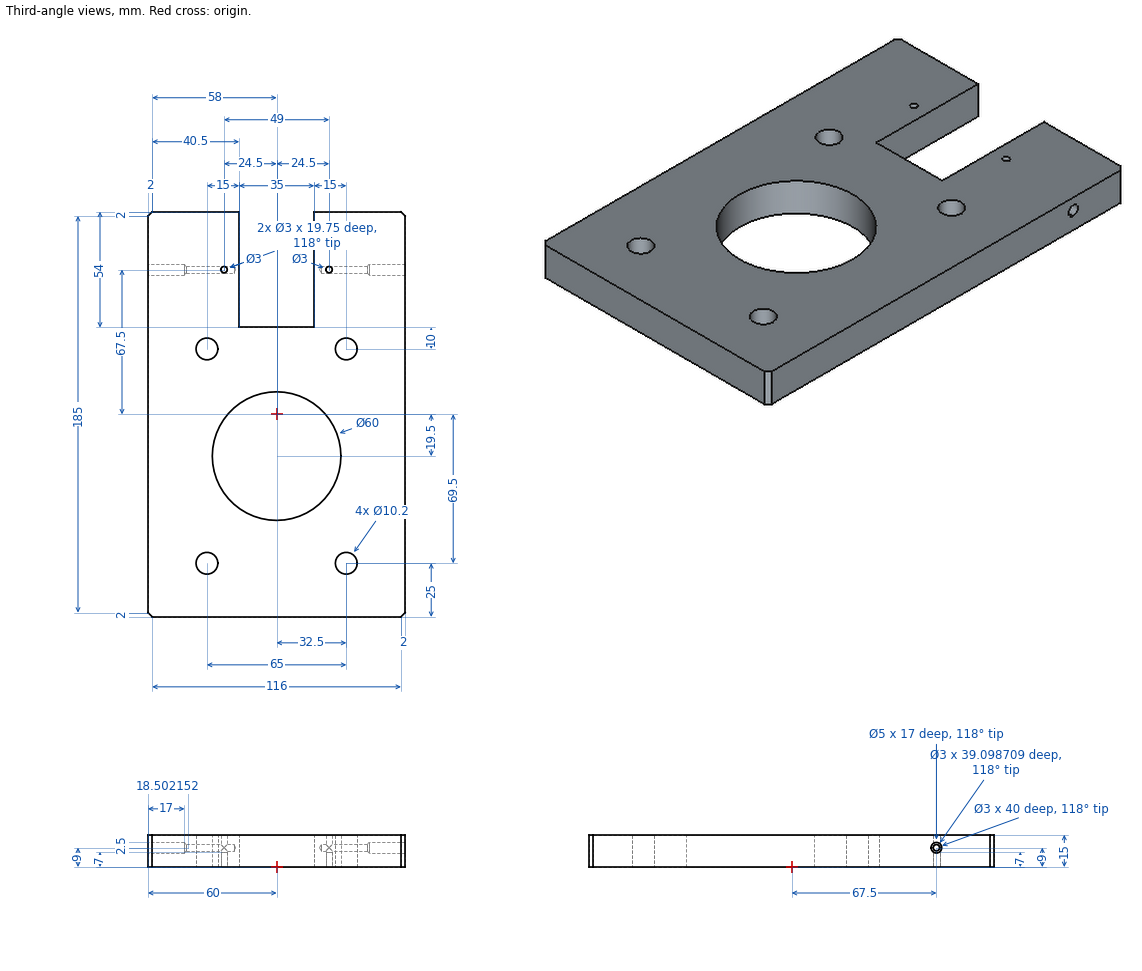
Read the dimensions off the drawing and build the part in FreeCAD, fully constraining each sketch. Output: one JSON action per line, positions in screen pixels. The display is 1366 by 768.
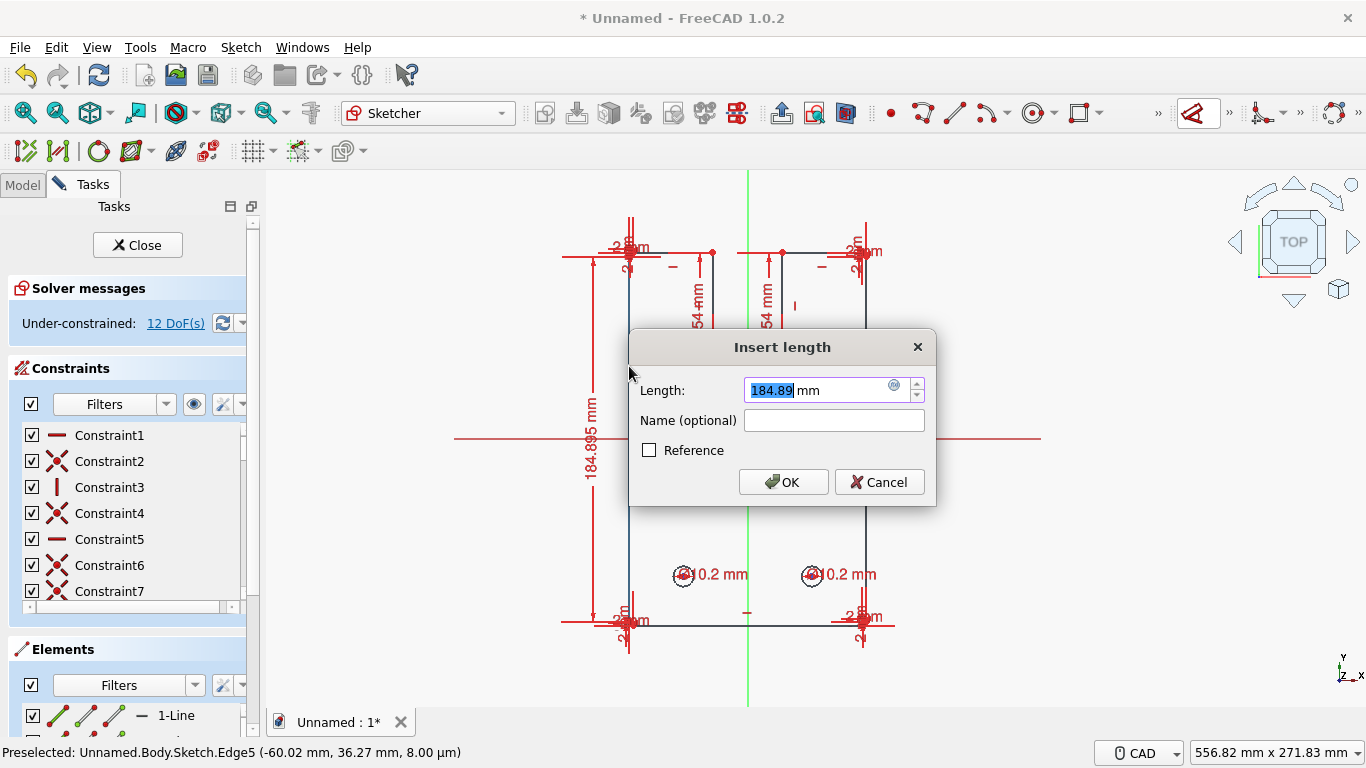
{"action": "type", "text": "185"}
{"action": "key", "text": "Return"}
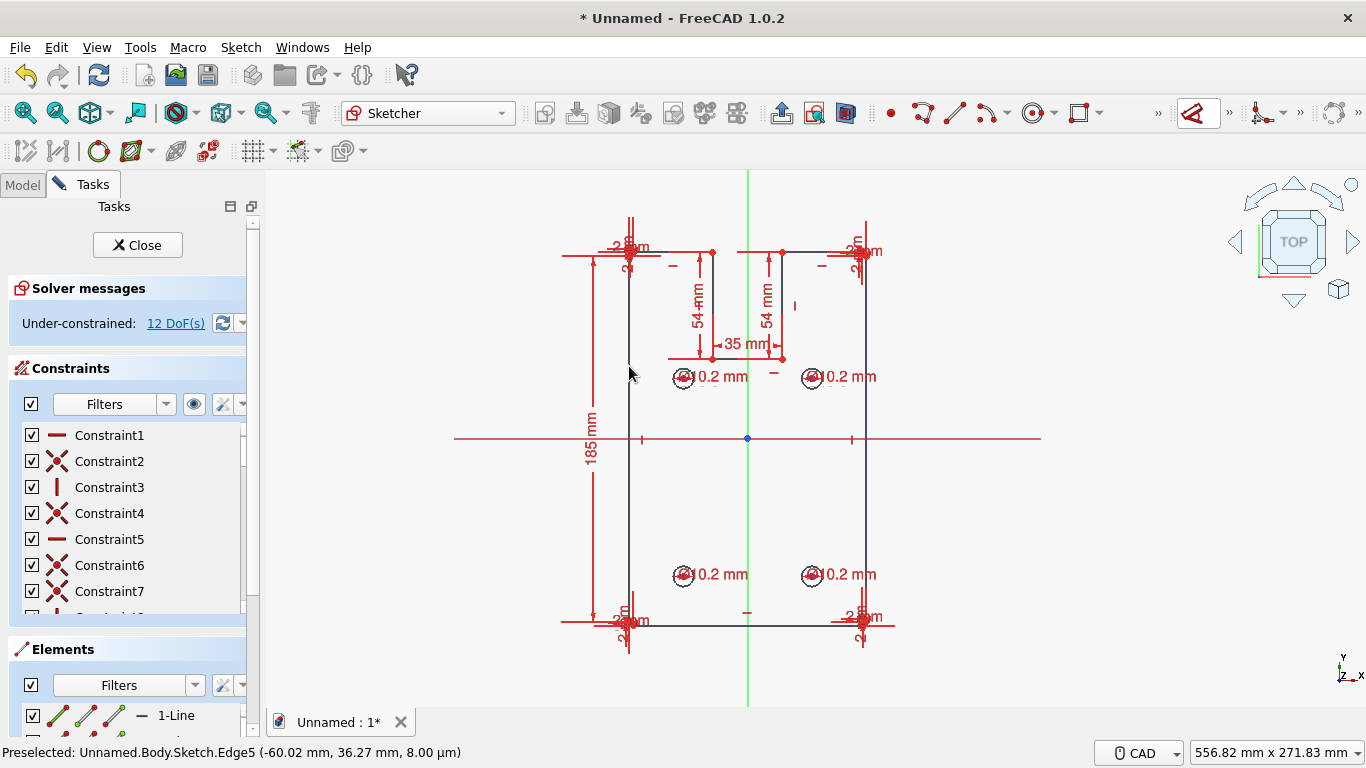
{"action": "left_click", "coordinate": [702, 626]}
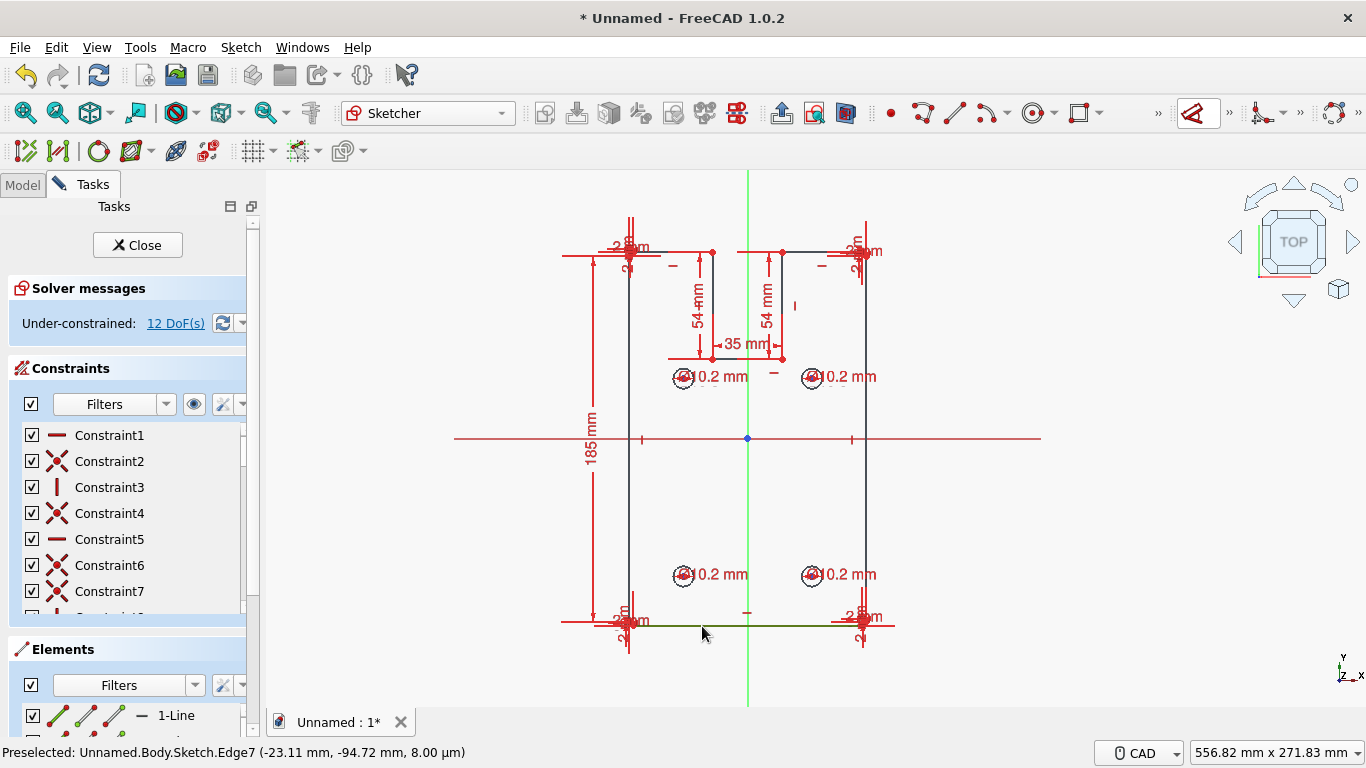
{"action": "key", "text": "l"}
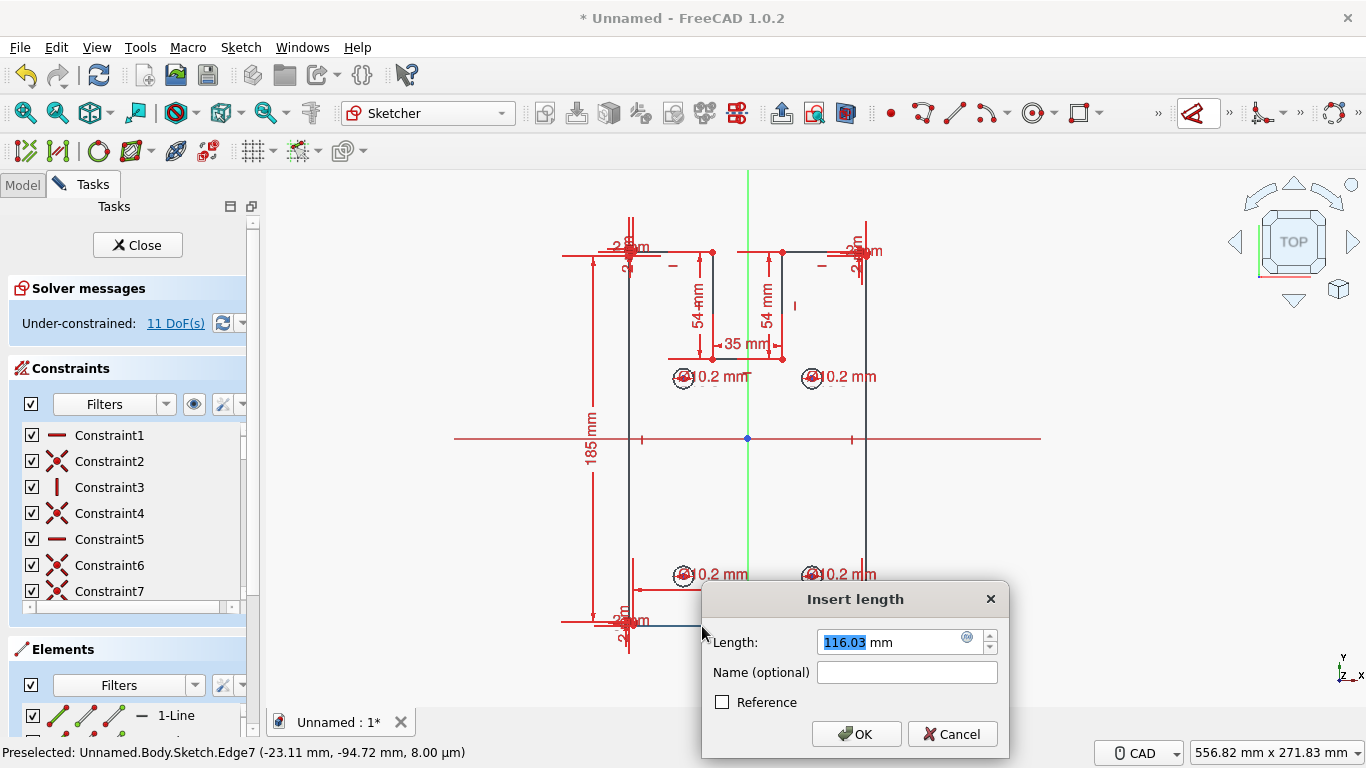
{"action": "type", "text": "116"}
{"action": "key", "text": "Return"}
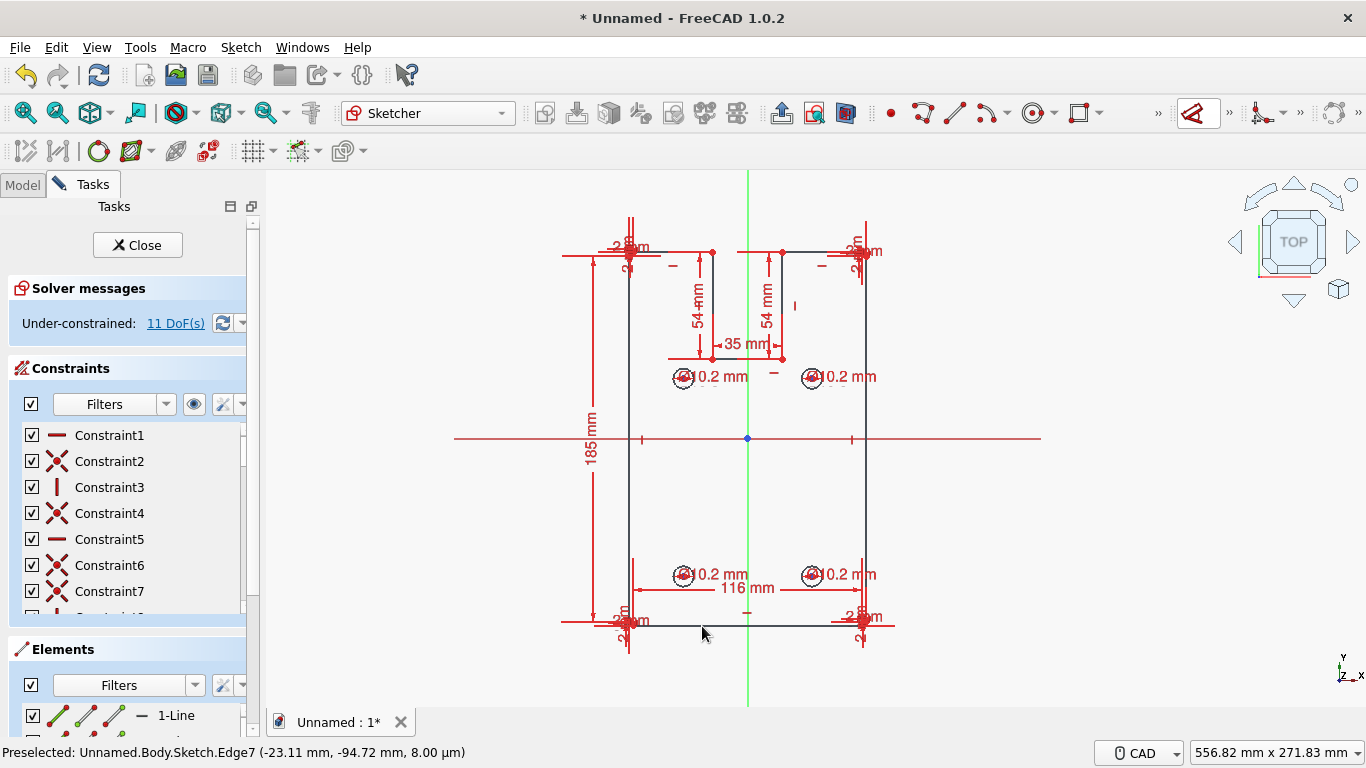
{"action": "scroll", "coordinate": [633, 252], "scroll_direction": "up", "scroll_amount": 4}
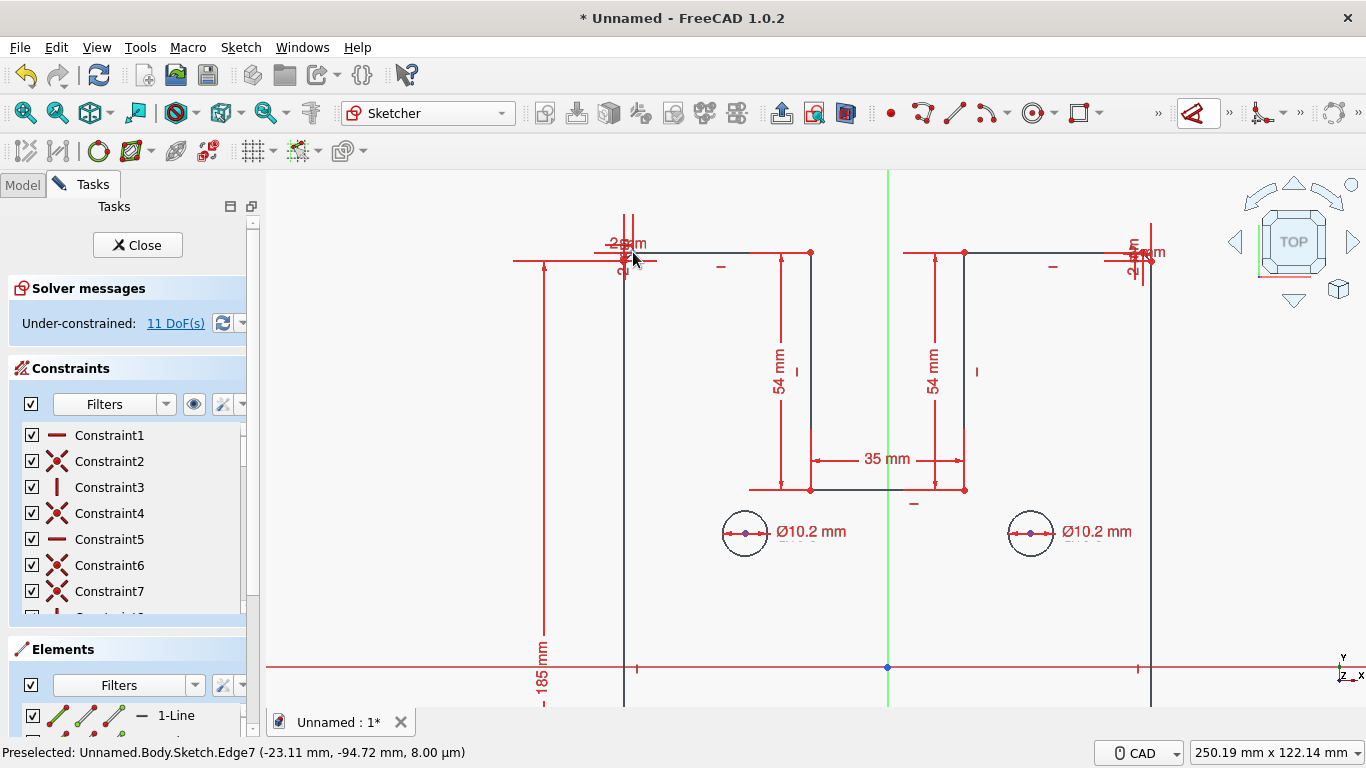
{"action": "left_click", "coordinate": [633, 253]}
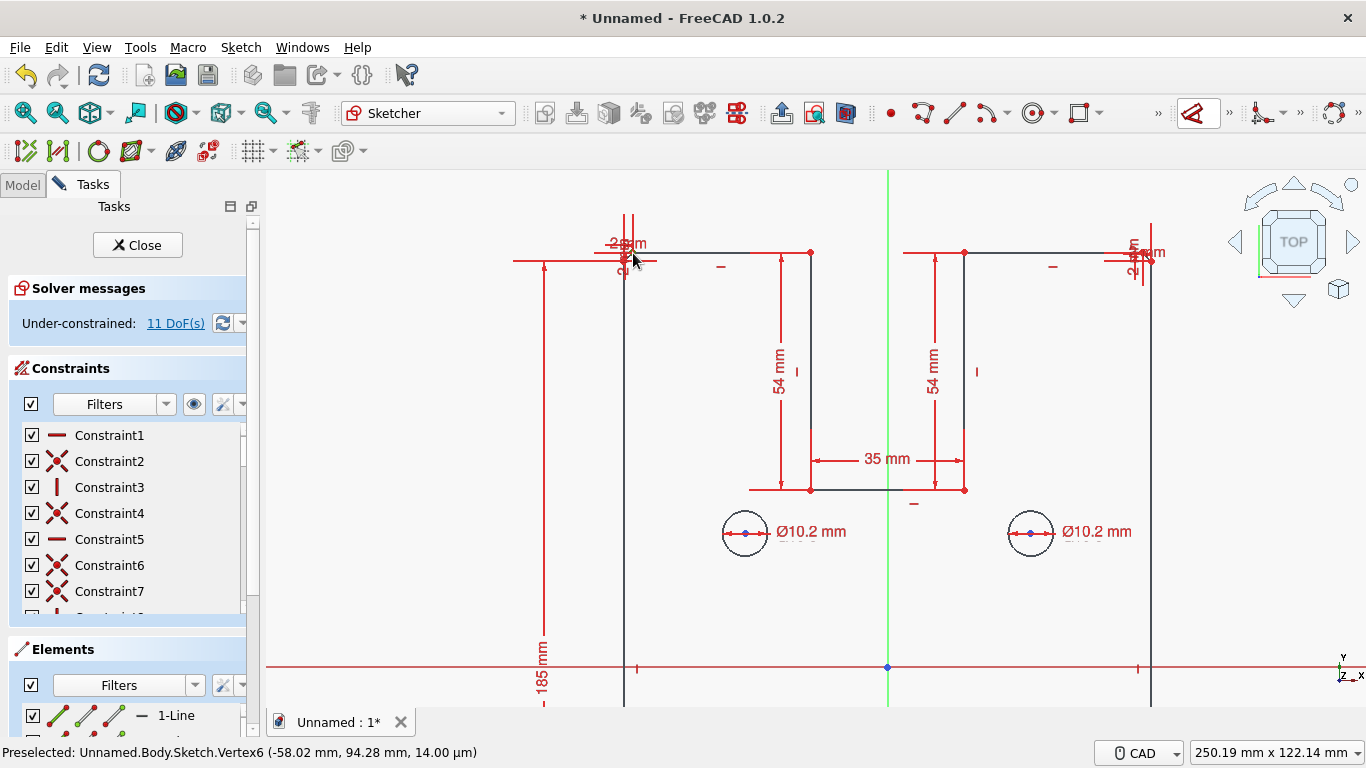
{"action": "left_click", "coordinate": [1214, 114]}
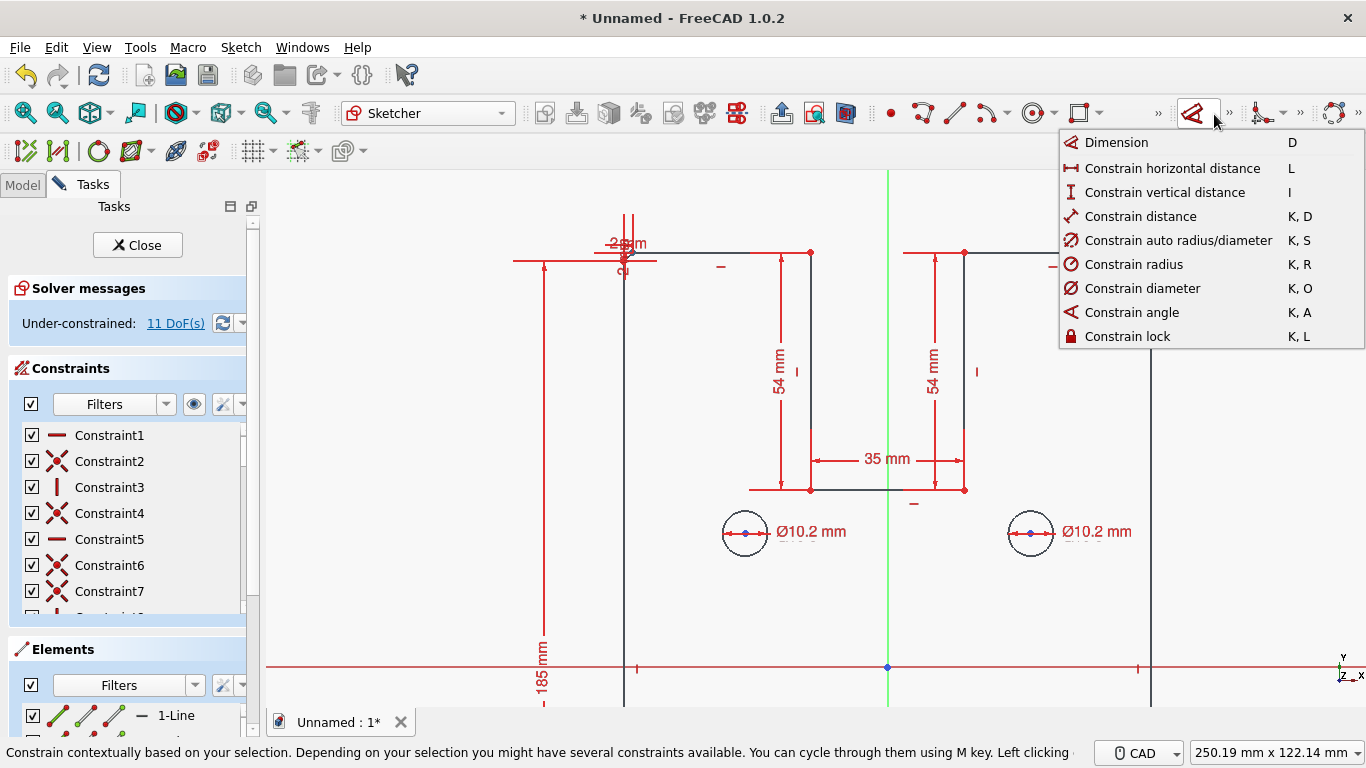
{"action": "left_click", "coordinate": [1212, 168]}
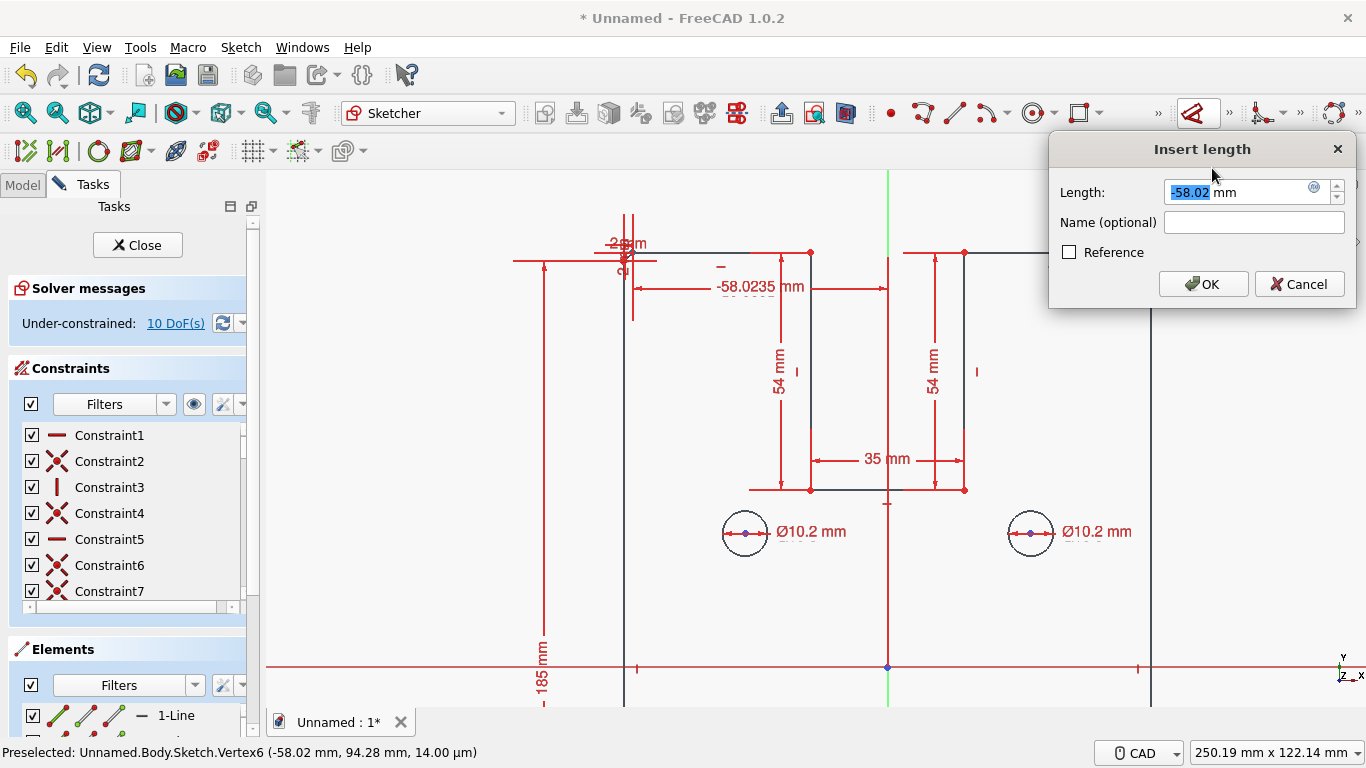
{"action": "type", "text": "-58"}
{"action": "key", "text": "Return"}